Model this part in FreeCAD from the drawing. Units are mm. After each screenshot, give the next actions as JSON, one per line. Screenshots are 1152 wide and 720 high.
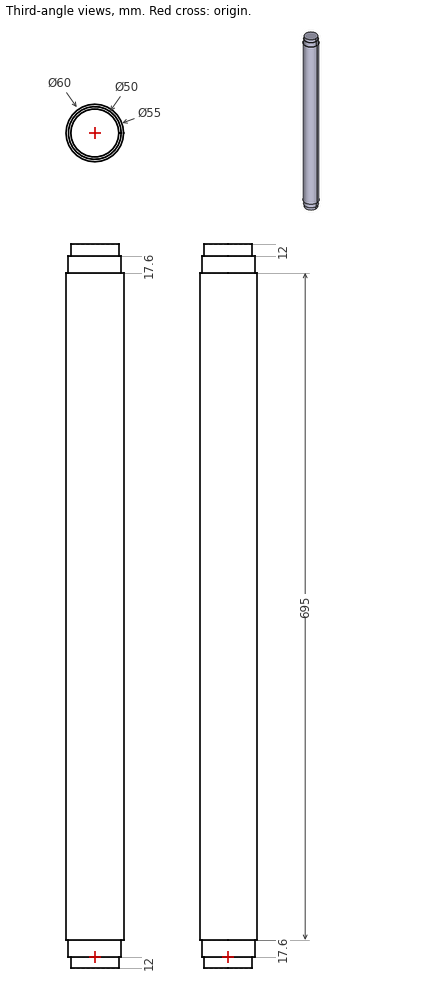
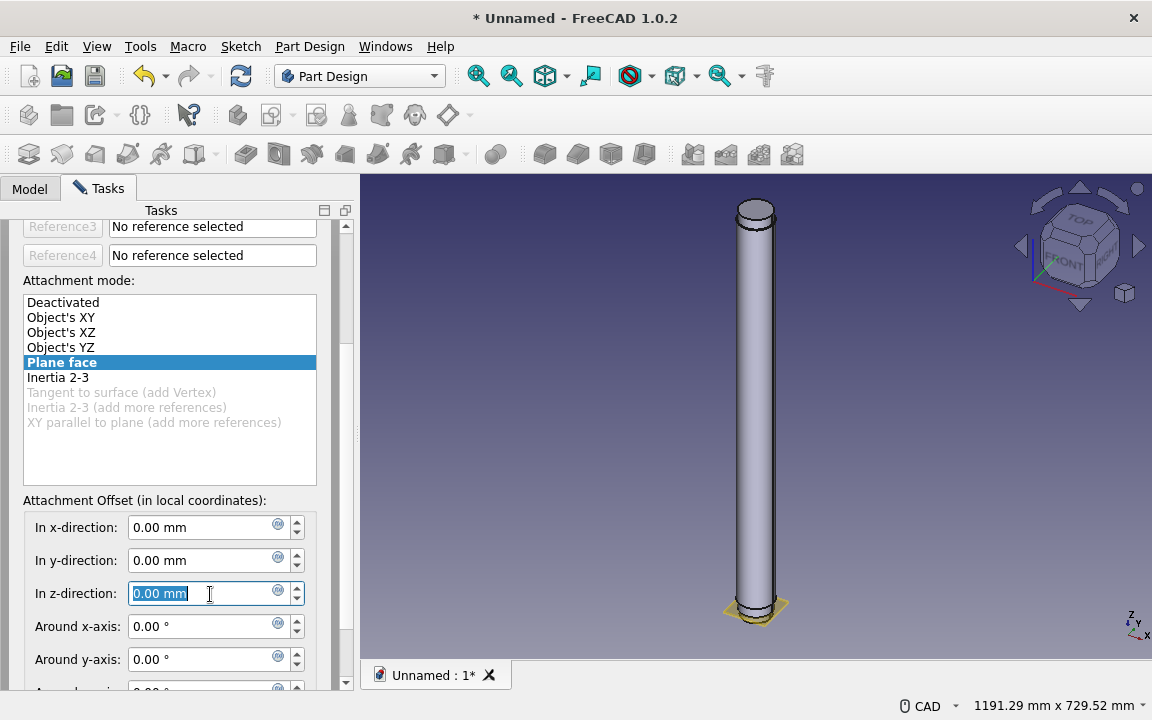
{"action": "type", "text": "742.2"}
{"action": "key", "text": "Tab"}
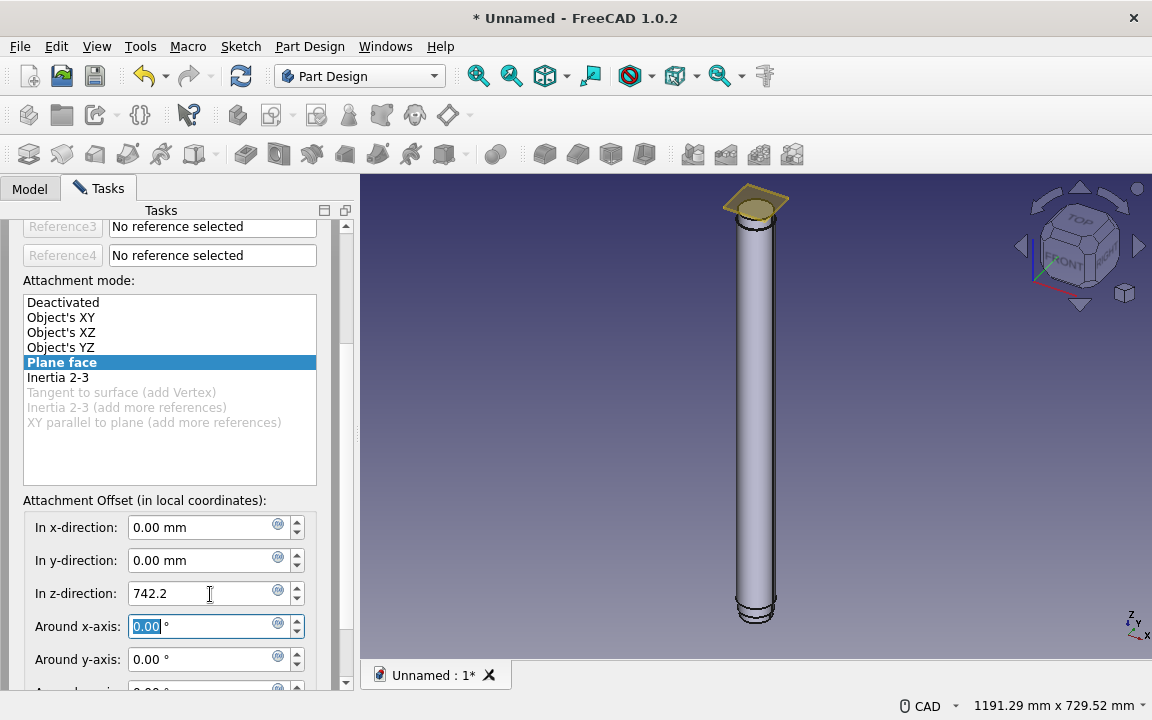
{"action": "scroll", "coordinate": [346, 455], "scroll_direction": "up", "scroll_amount": 4}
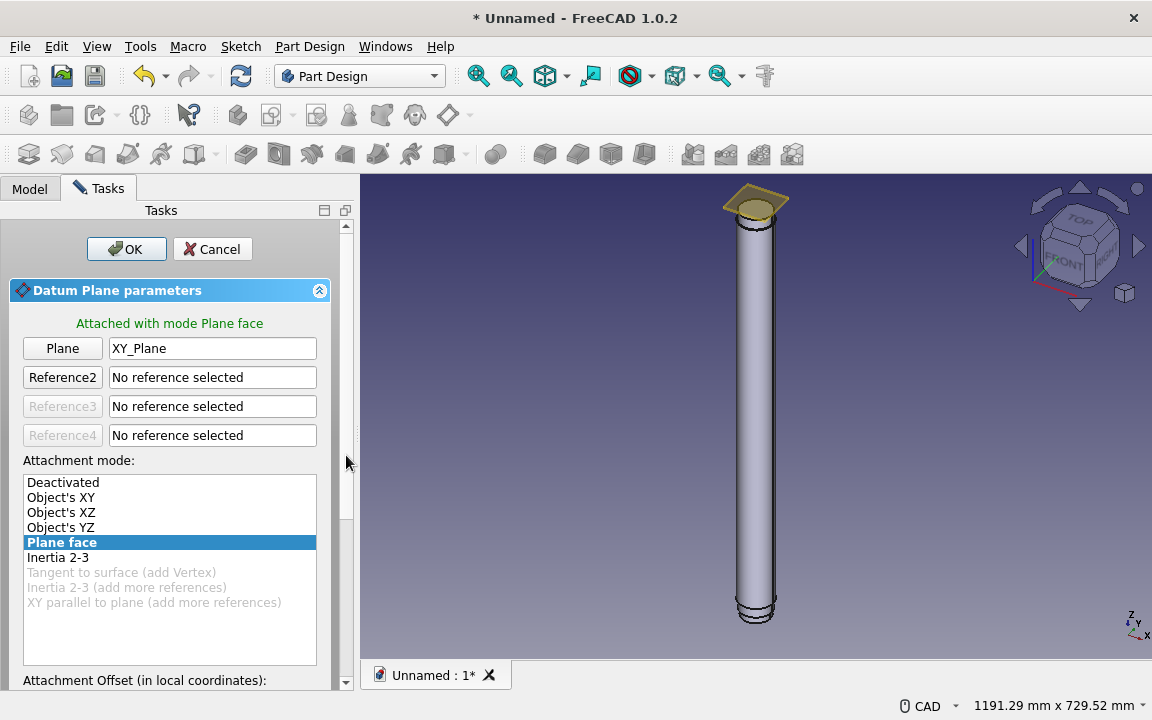
{"action": "left_click", "coordinate": [127, 249]}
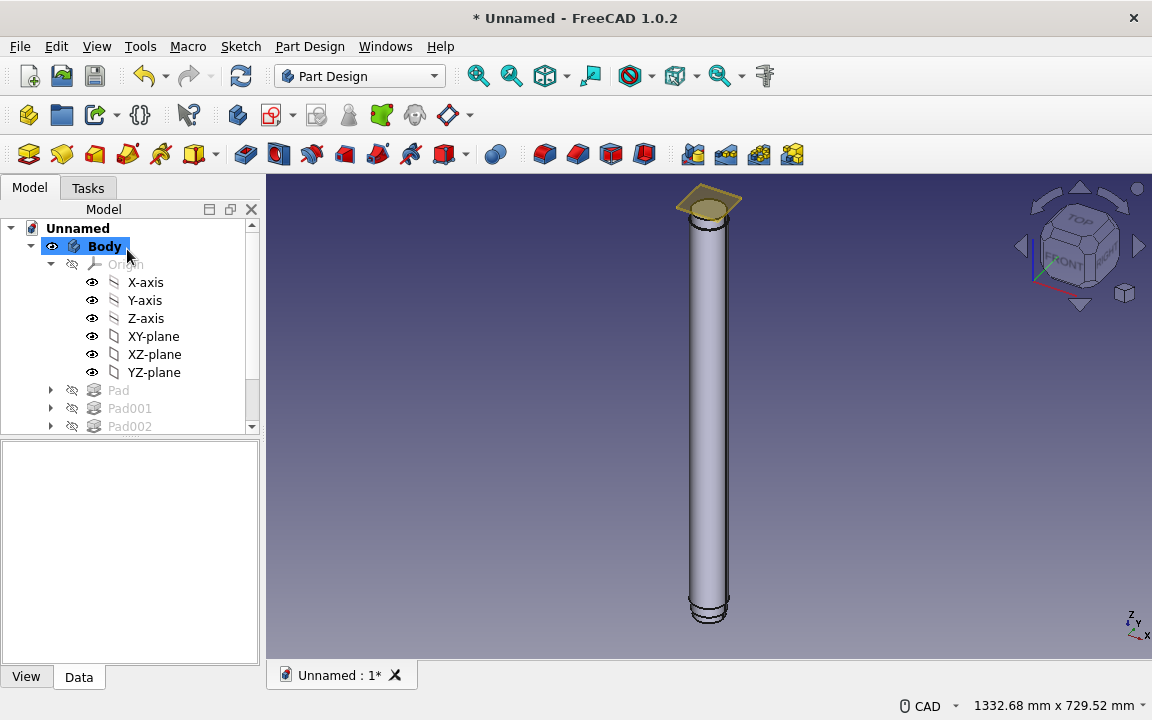
{"action": "scroll", "coordinate": [101, 332], "scroll_direction": "down", "scroll_amount": 3}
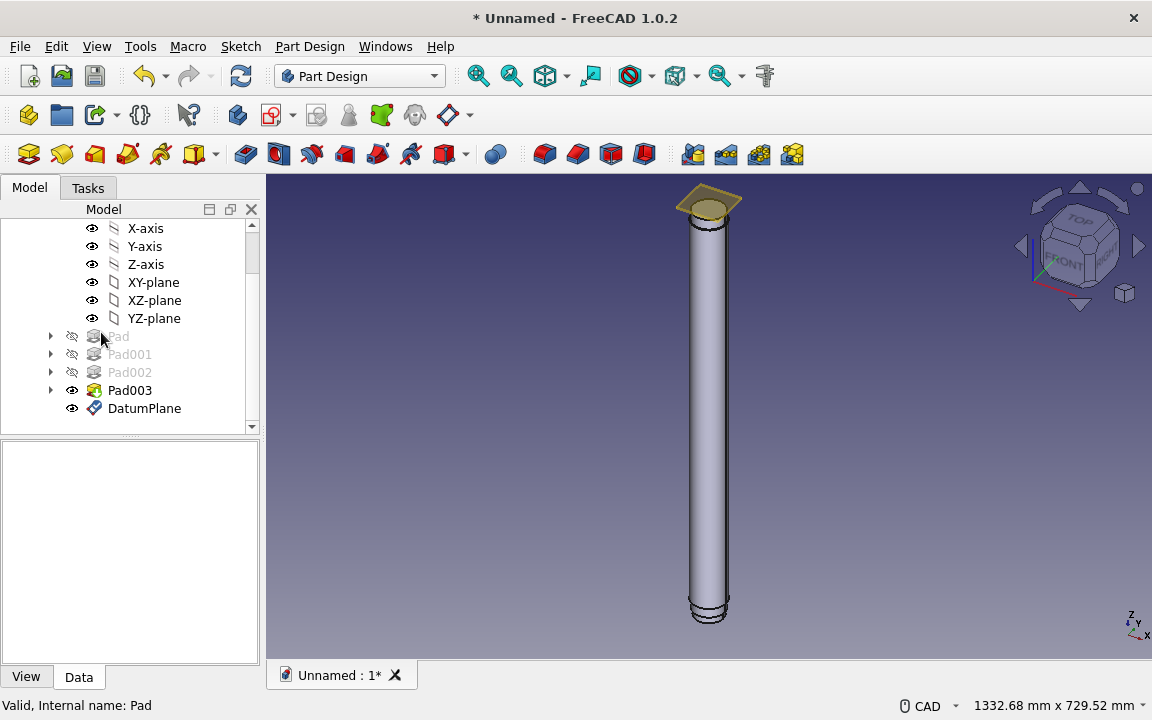
{"action": "left_click", "coordinate": [117, 408]}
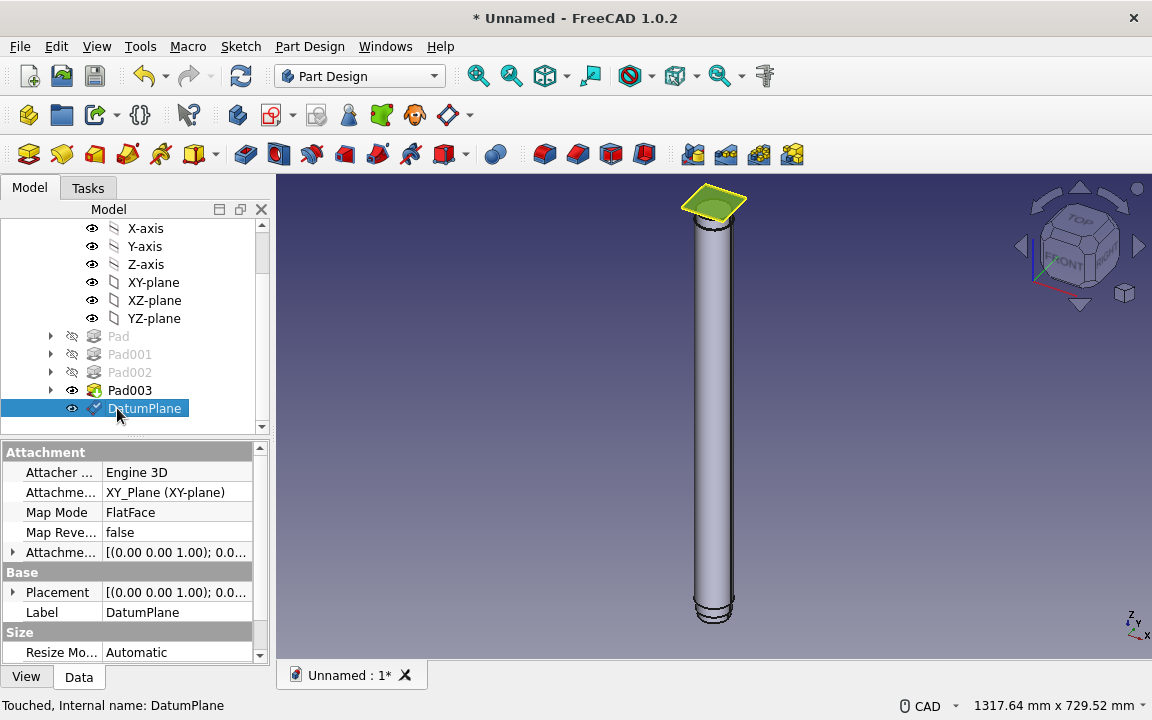
{"action": "left_click", "coordinate": [270, 116]}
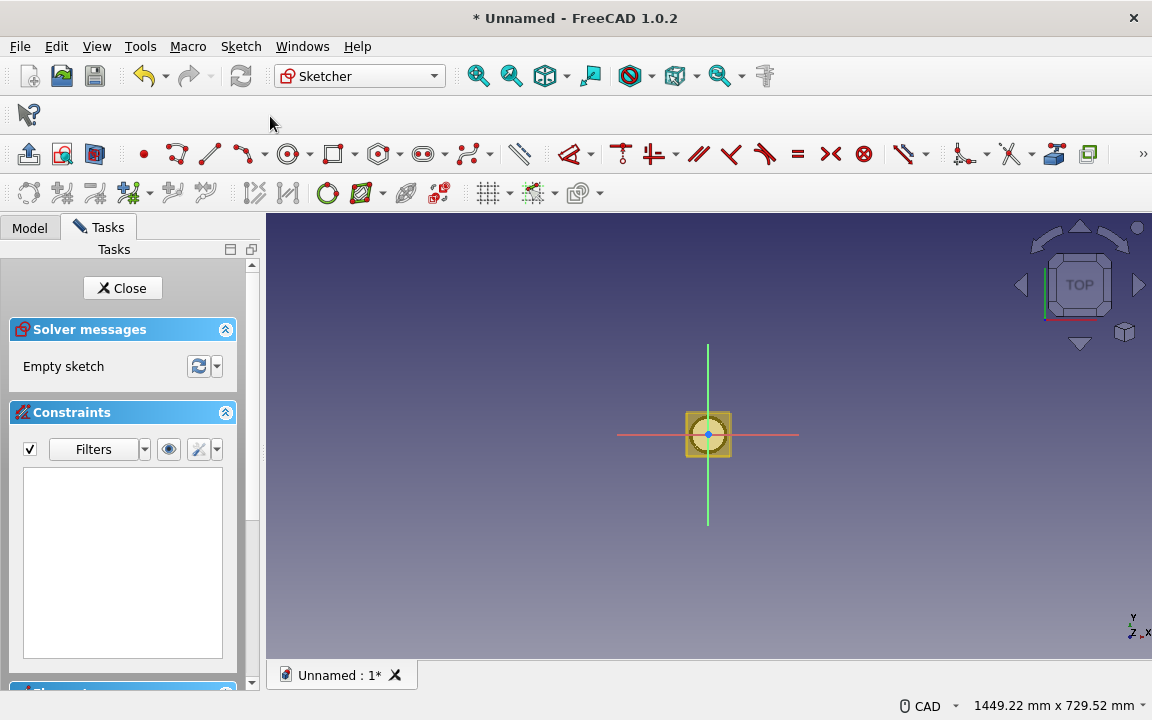
{"action": "scroll", "coordinate": [717, 435], "scroll_direction": "up", "scroll_amount": 11}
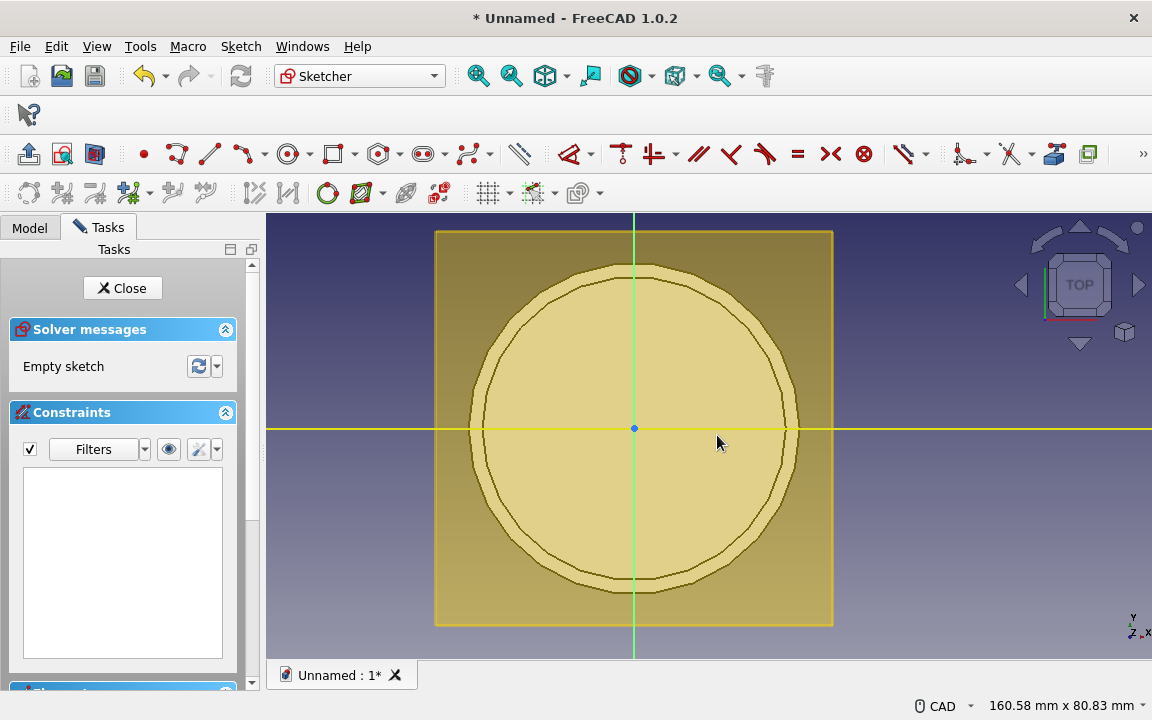
{"action": "left_click", "coordinate": [288, 154]}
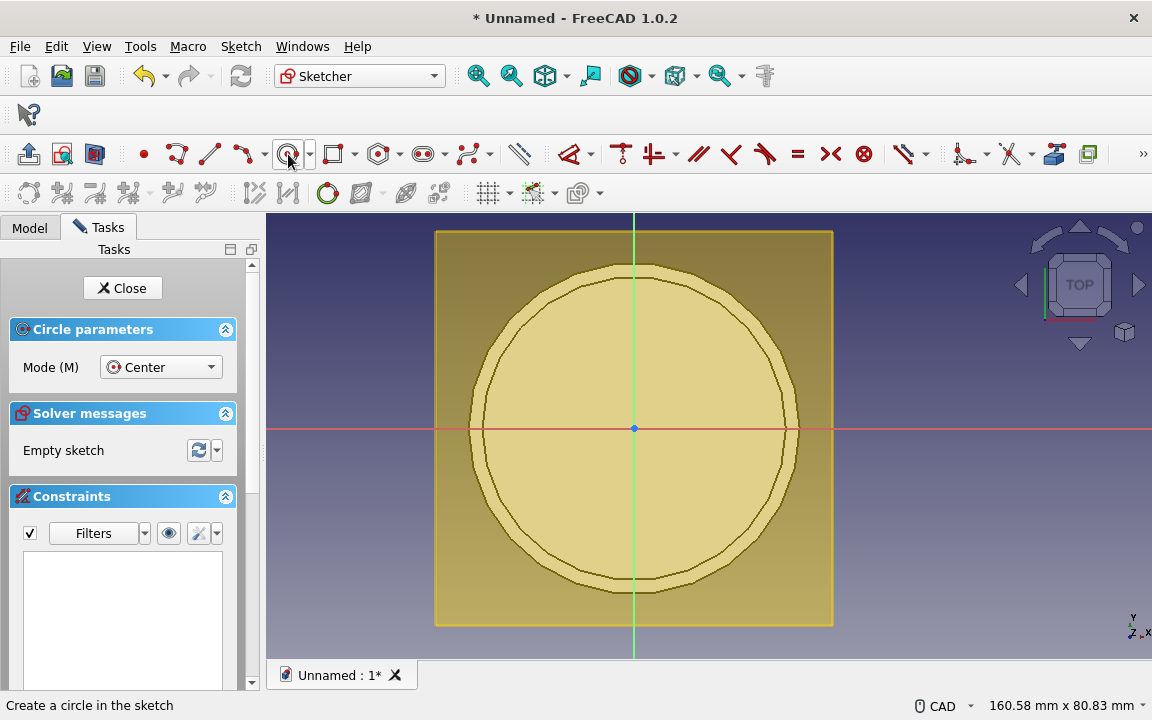
{"action": "left_click", "coordinate": [634, 429]}
{"action": "mouse_move", "coordinate": [732, 331]}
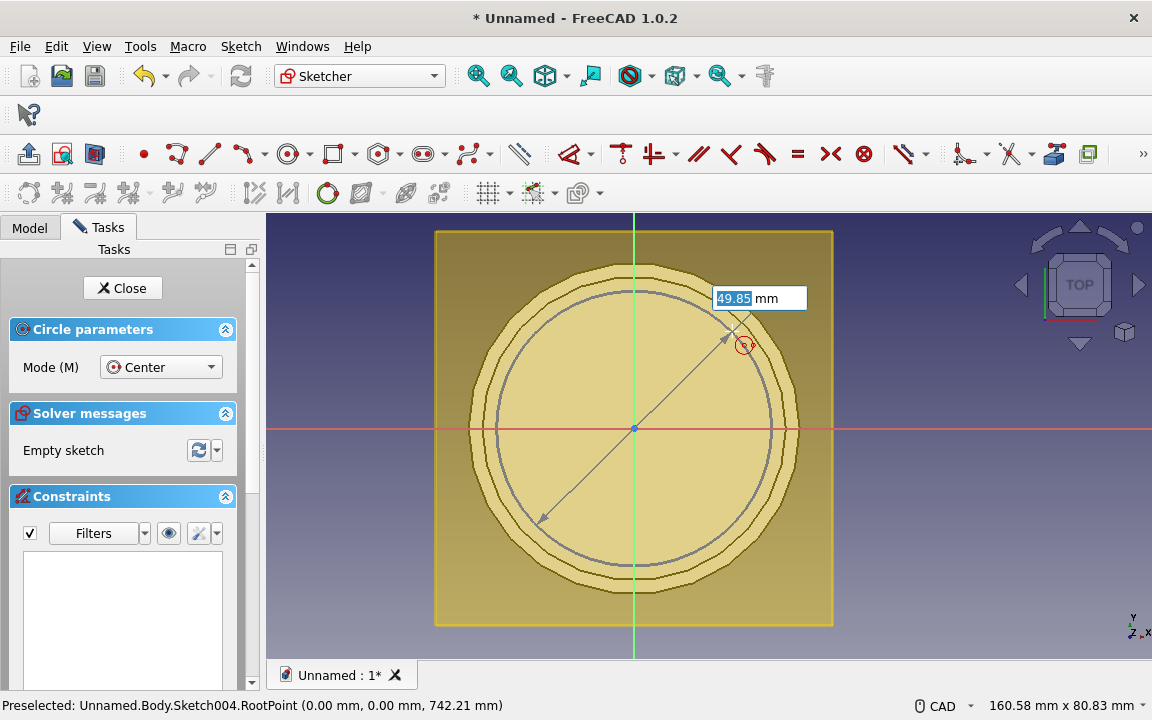
{"action": "type", "text": "50"}
{"action": "key", "text": "Return"}
{"action": "key", "text": "Escape"}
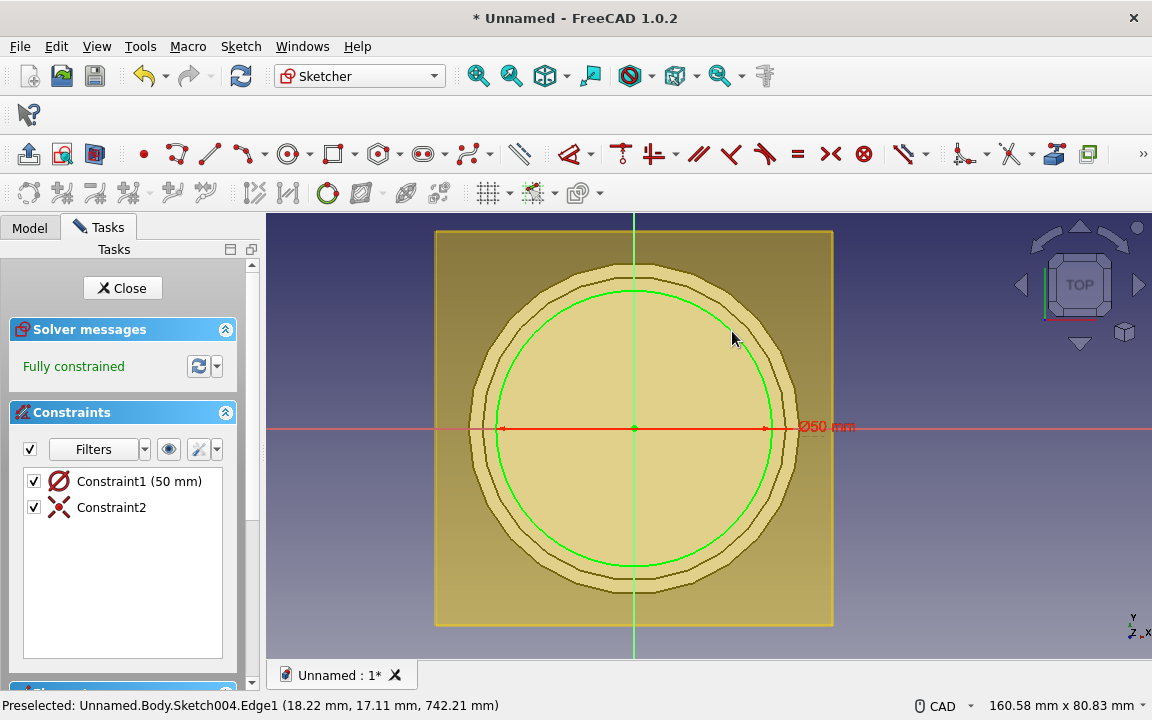
{"action": "left_click", "coordinate": [123, 288]}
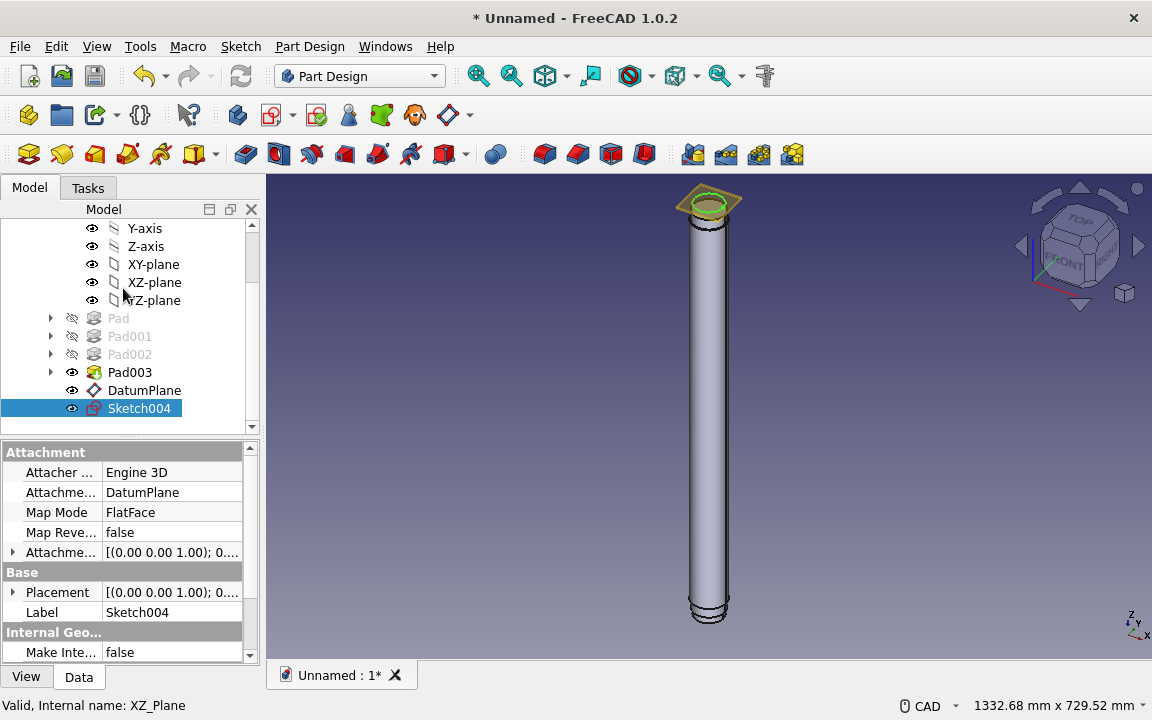
{"action": "left_click", "coordinate": [29, 154]}